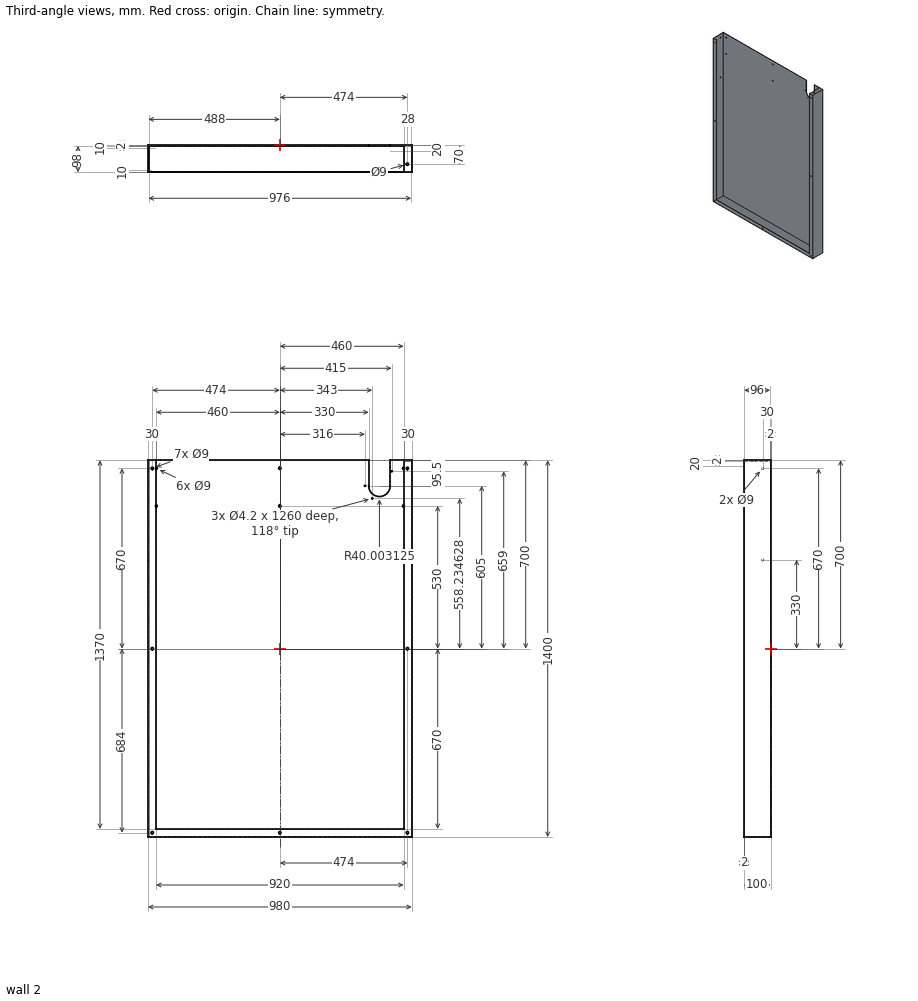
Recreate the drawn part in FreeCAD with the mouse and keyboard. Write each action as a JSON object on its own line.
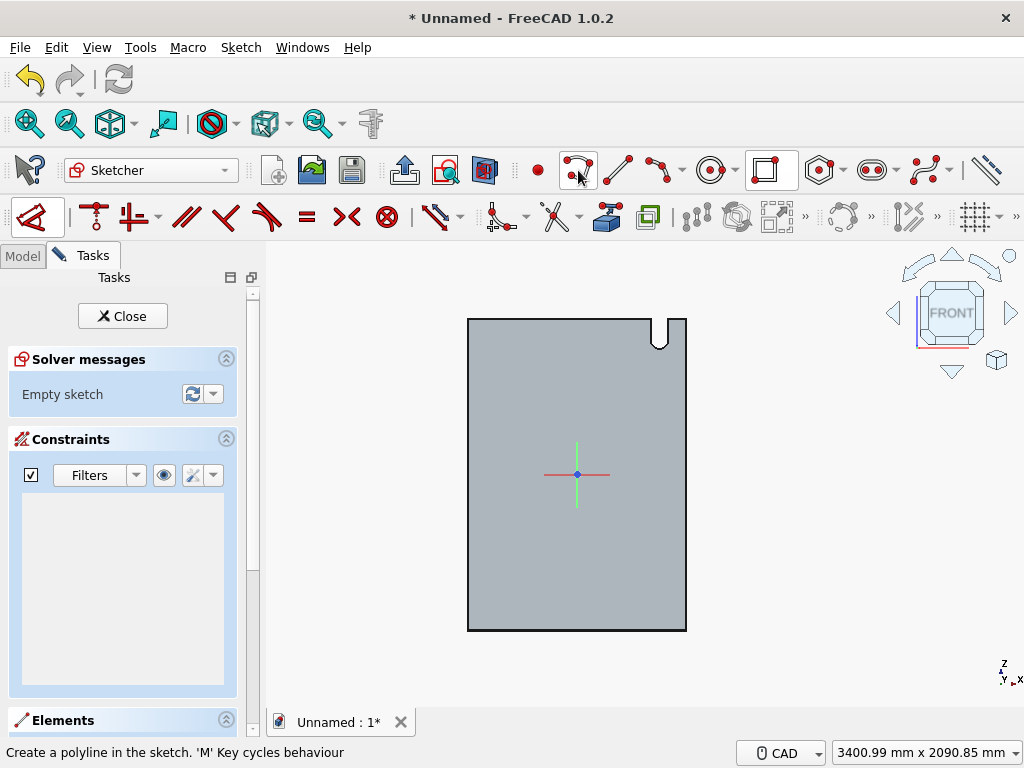
{"action": "left_click", "coordinate": [680, 624]}
{"action": "left_click", "coordinate": [475, 624]}
{"action": "left_click", "coordinate": [475, 319]}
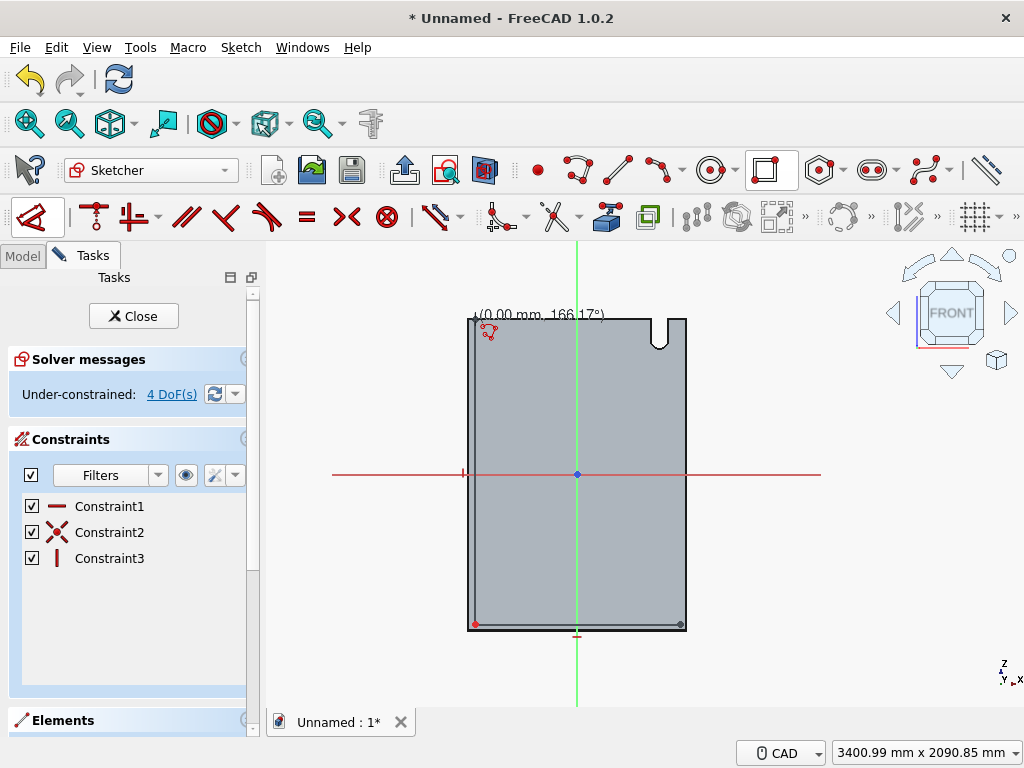
{"action": "scroll", "coordinate": [468, 319], "scroll_direction": "up", "scroll_amount": 5}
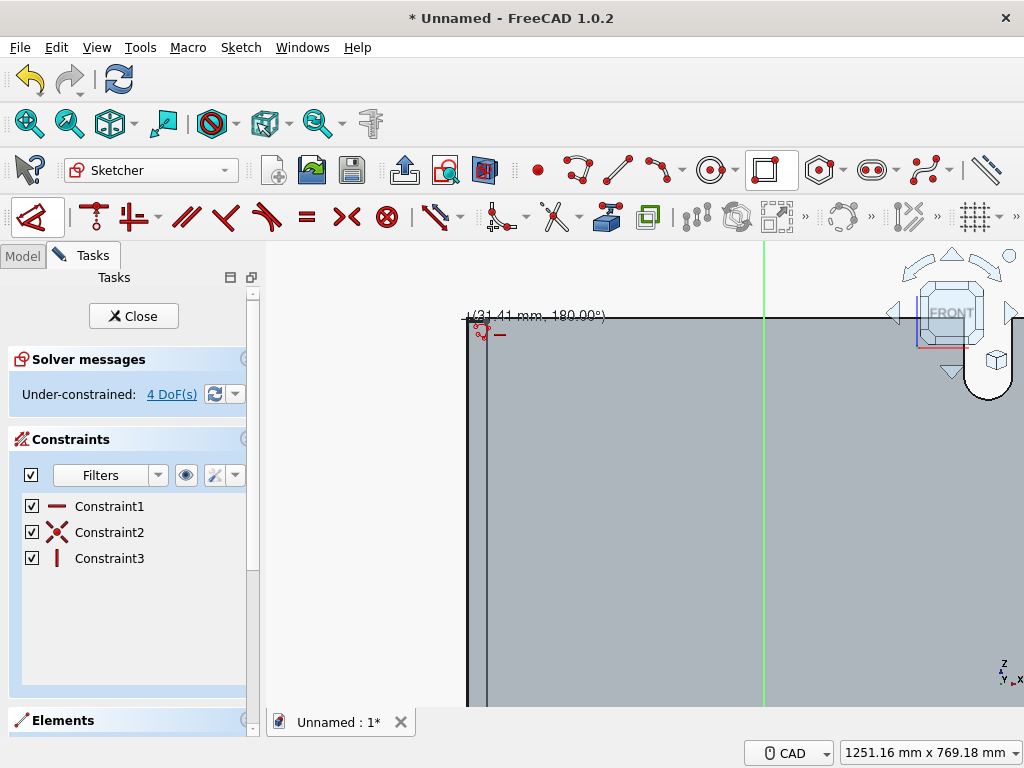
{"action": "left_click", "coordinate": [467, 319]}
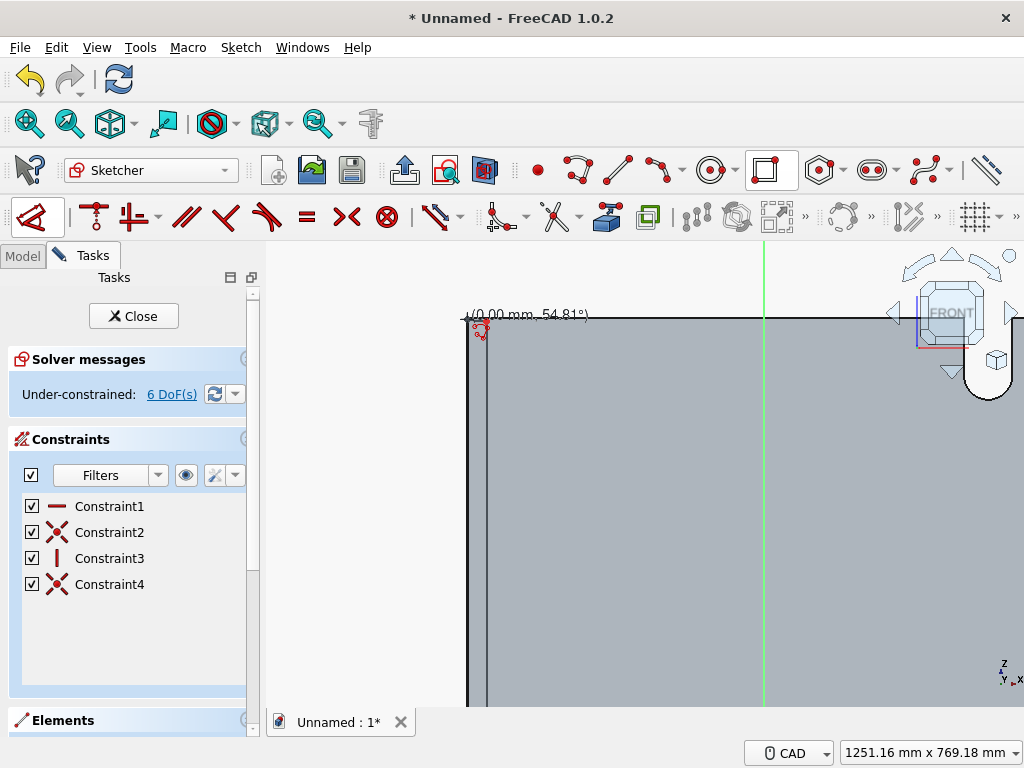
{"action": "scroll", "coordinate": [467, 318], "scroll_direction": "down", "scroll_amount": 5}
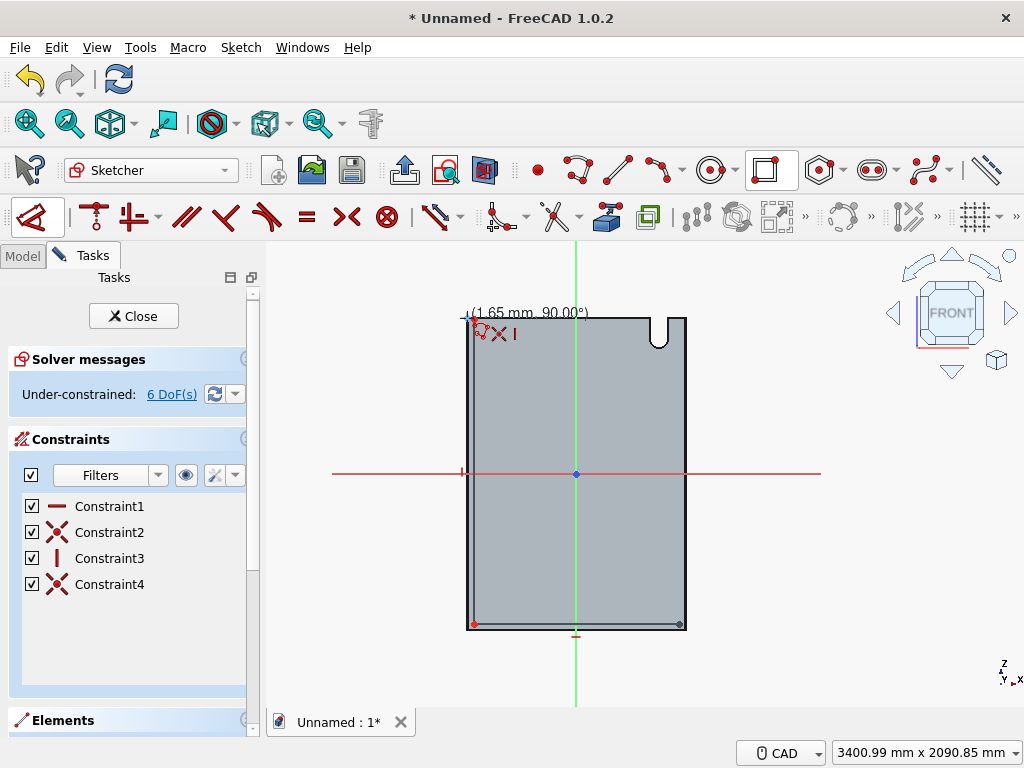
{"action": "scroll", "coordinate": [467, 630], "scroll_direction": "up", "scroll_amount": 3}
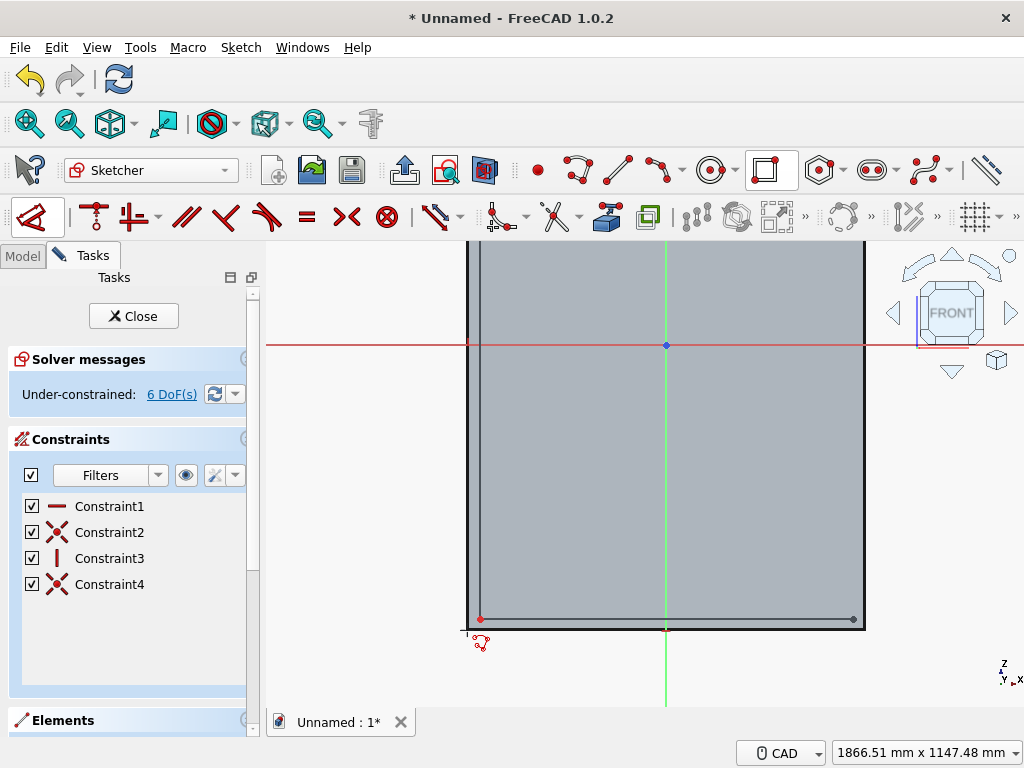
{"action": "left_click", "coordinate": [467, 630]}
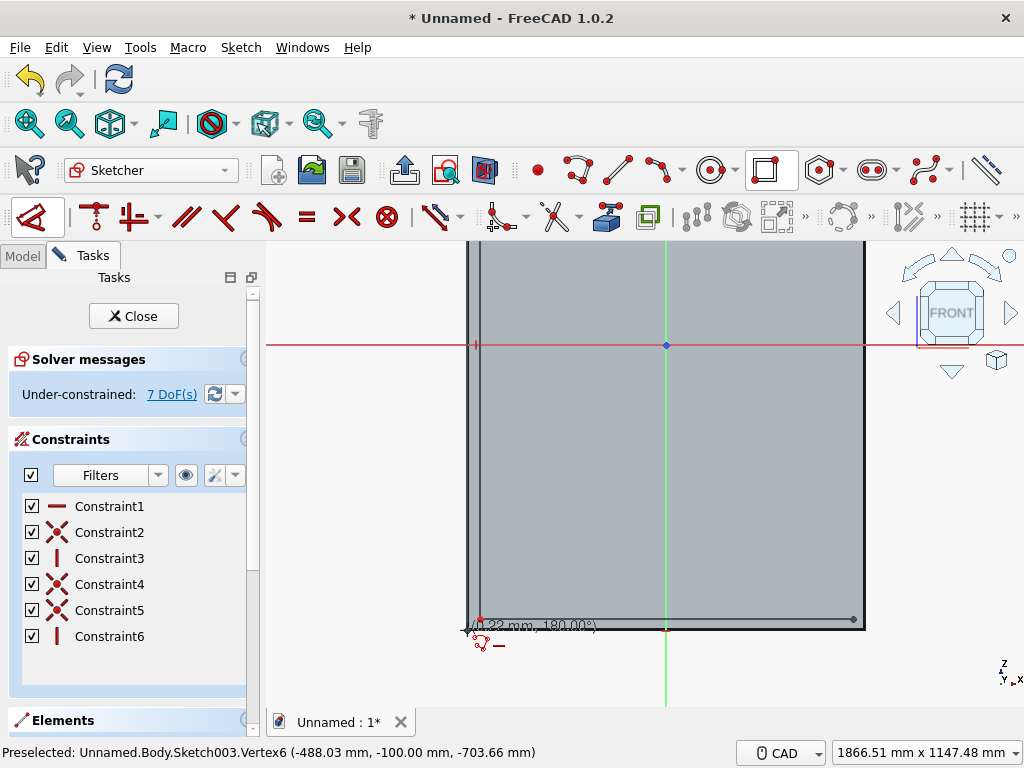
{"action": "scroll", "coordinate": [467, 631], "scroll_direction": "down", "scroll_amount": 3}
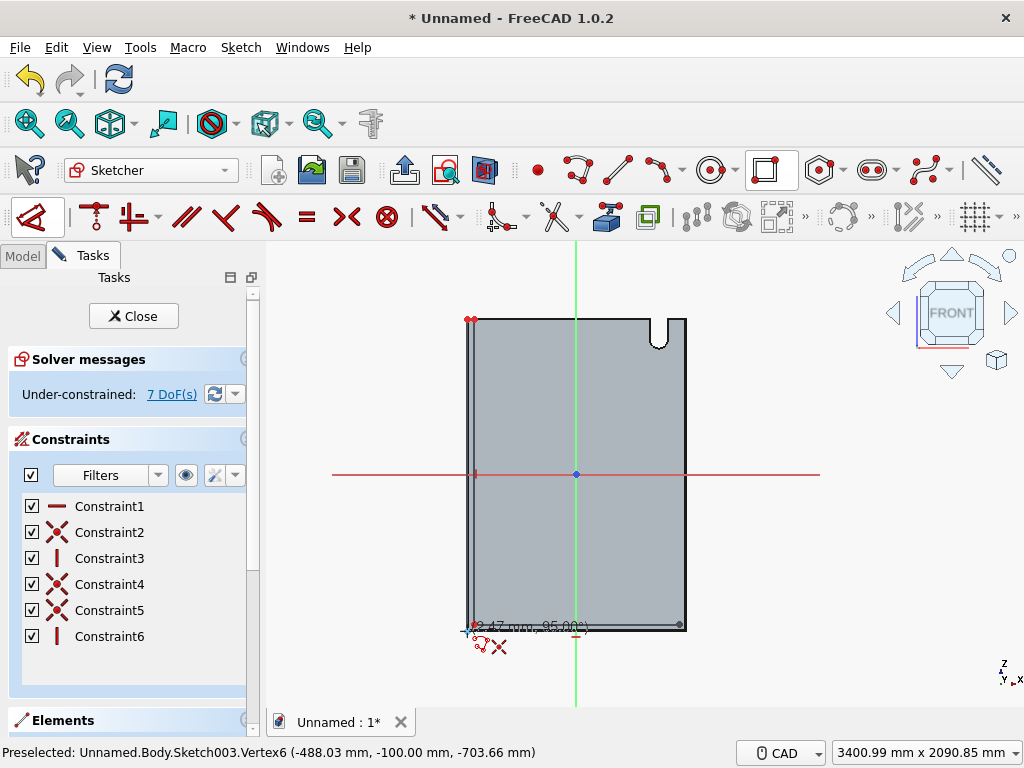
{"action": "scroll", "coordinate": [686, 631], "scroll_direction": "up", "scroll_amount": 3}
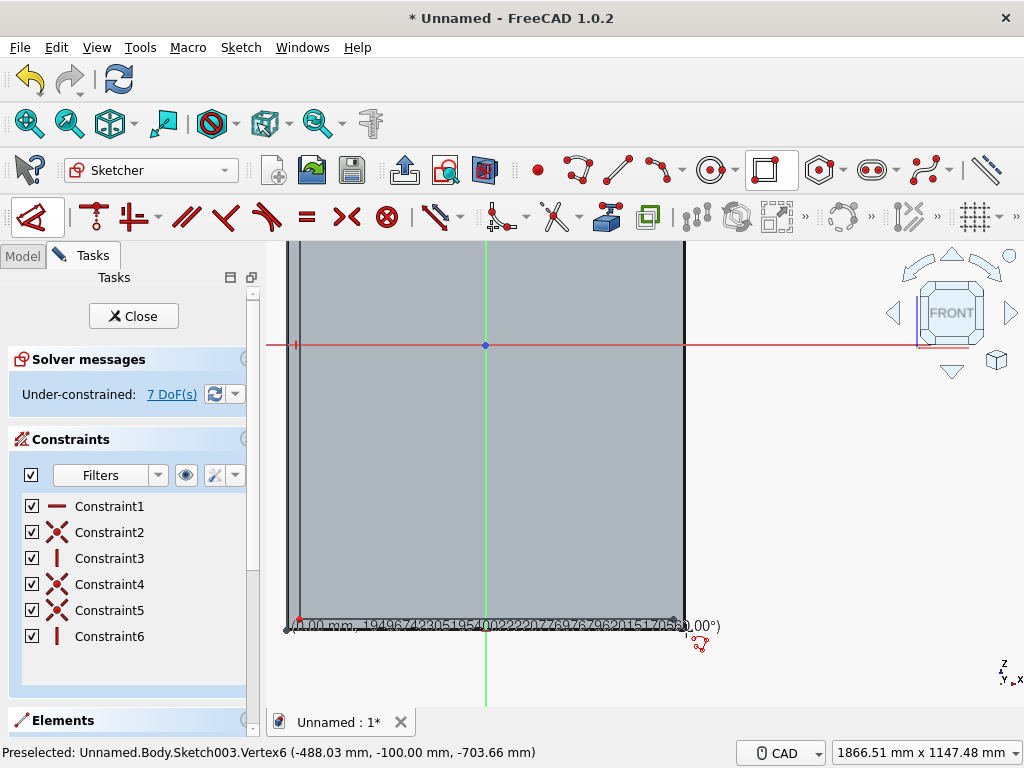
{"action": "left_click", "coordinate": [685, 630]}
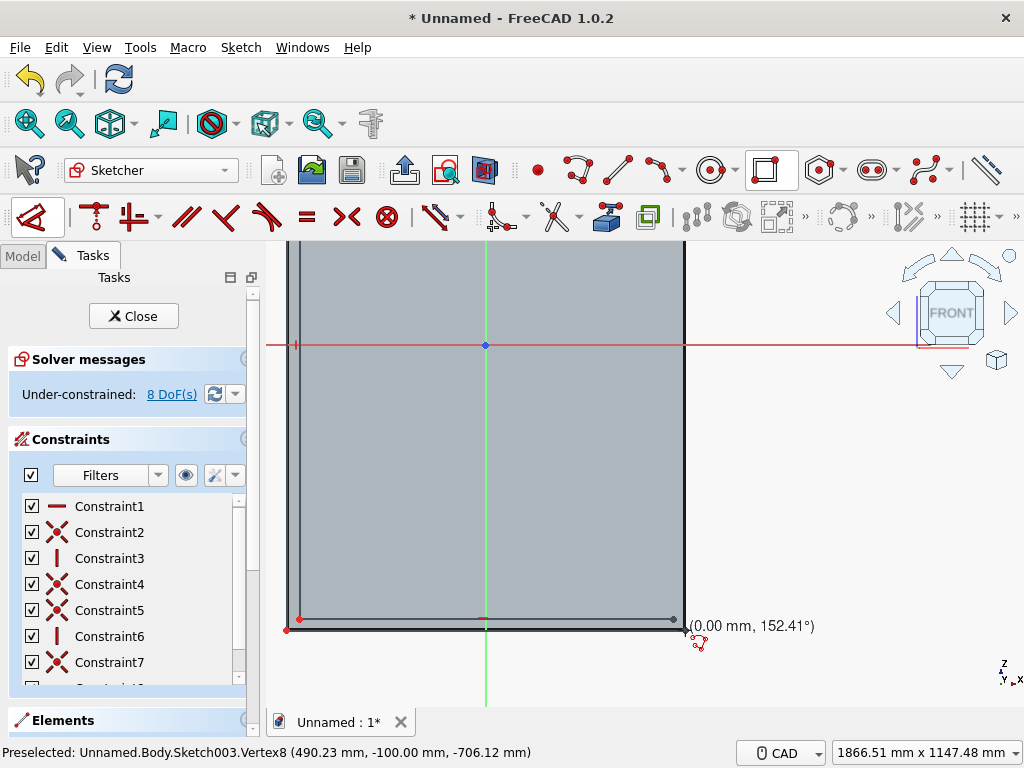
{"action": "scroll", "coordinate": [687, 631], "scroll_direction": "down", "scroll_amount": 3}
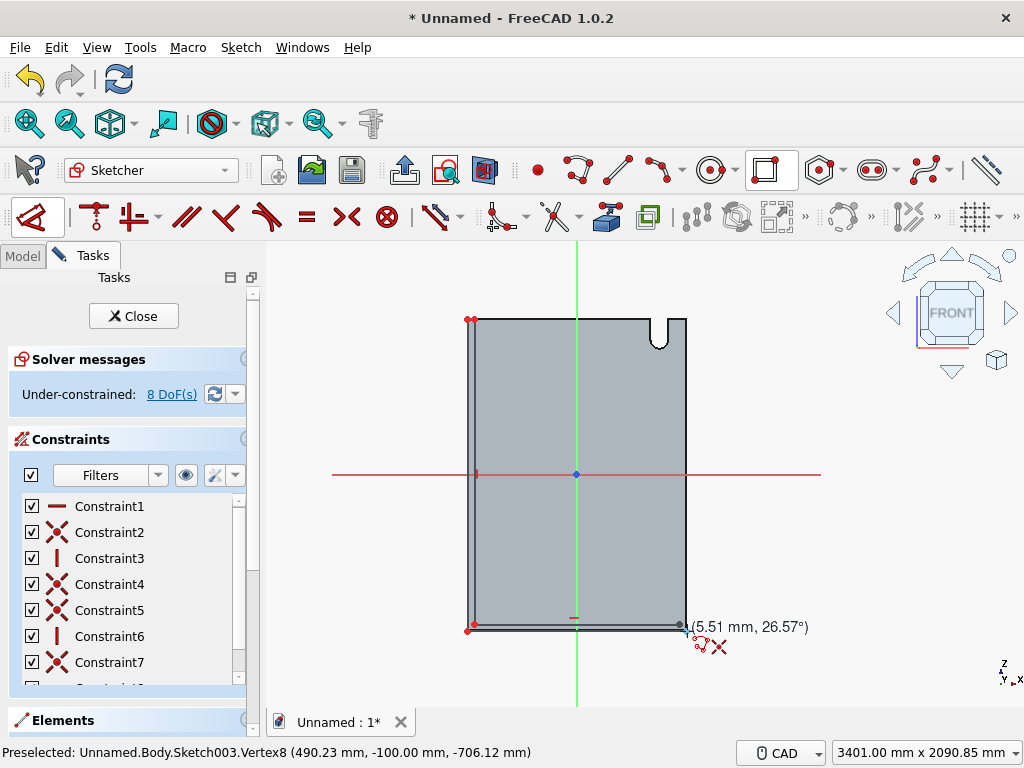
{"action": "left_click", "coordinate": [686, 319]}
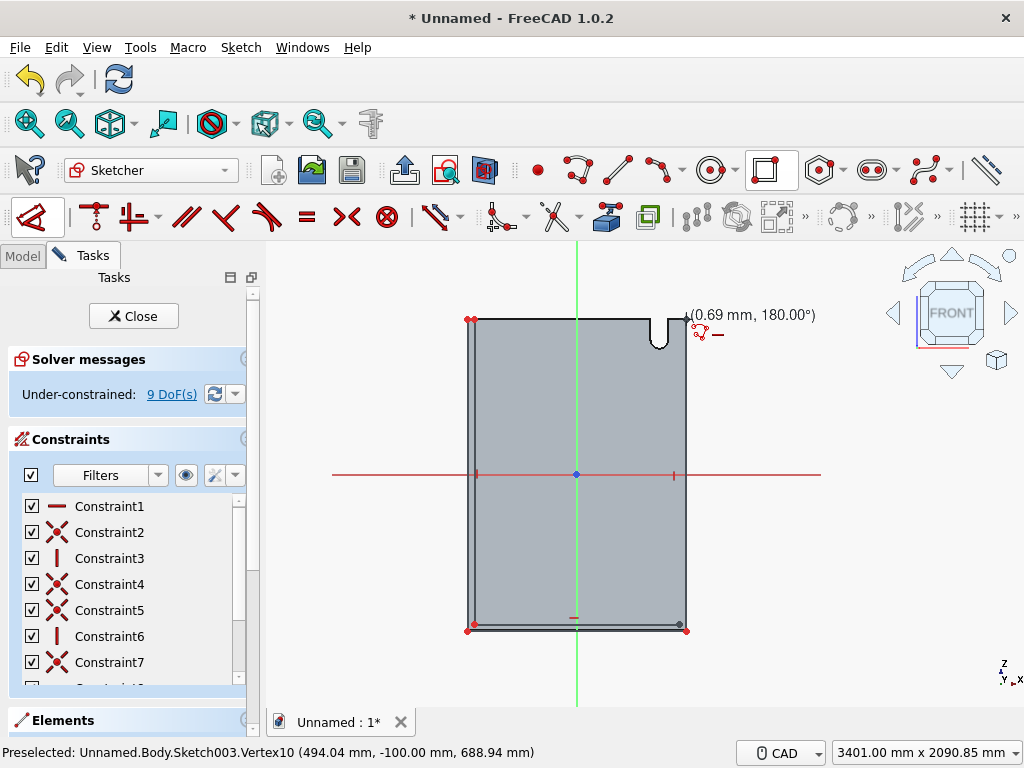
{"action": "scroll", "coordinate": [679, 319], "scroll_direction": "up", "scroll_amount": 5}